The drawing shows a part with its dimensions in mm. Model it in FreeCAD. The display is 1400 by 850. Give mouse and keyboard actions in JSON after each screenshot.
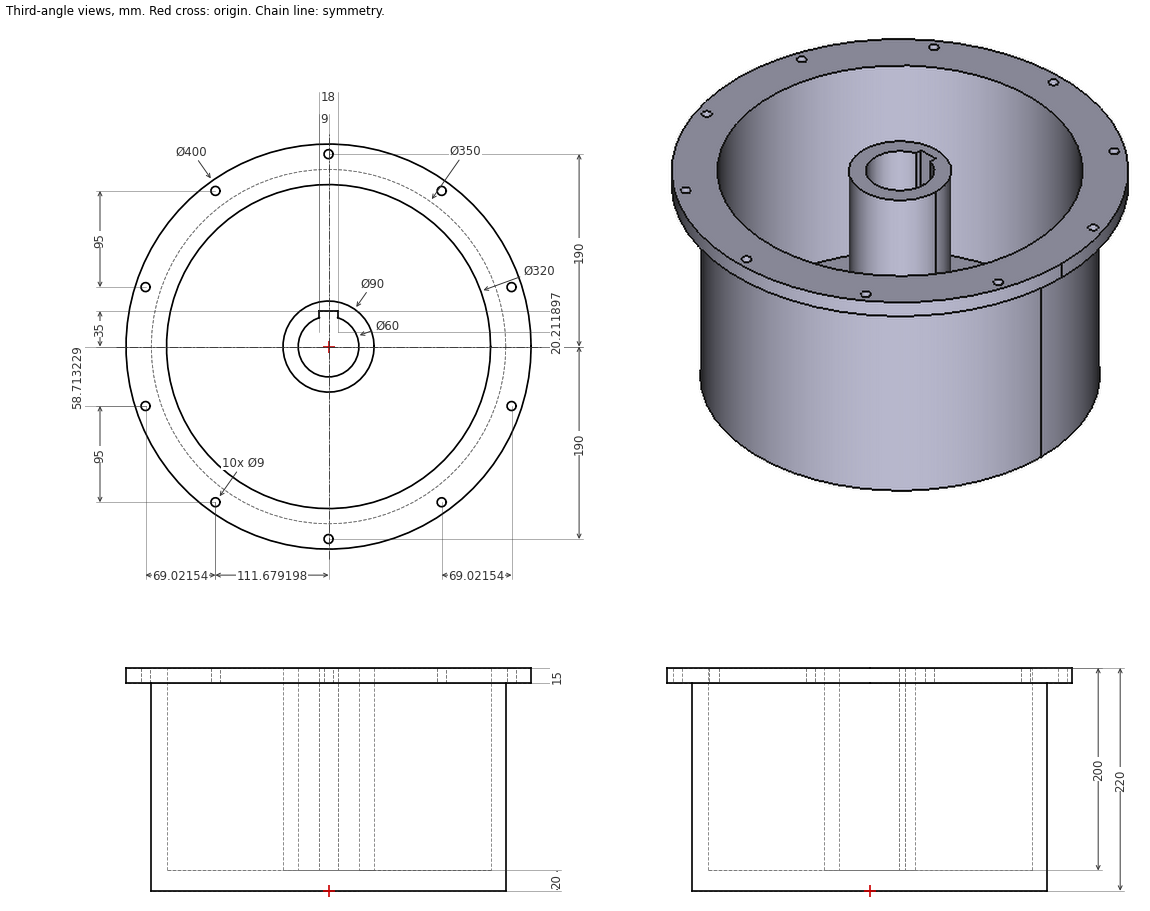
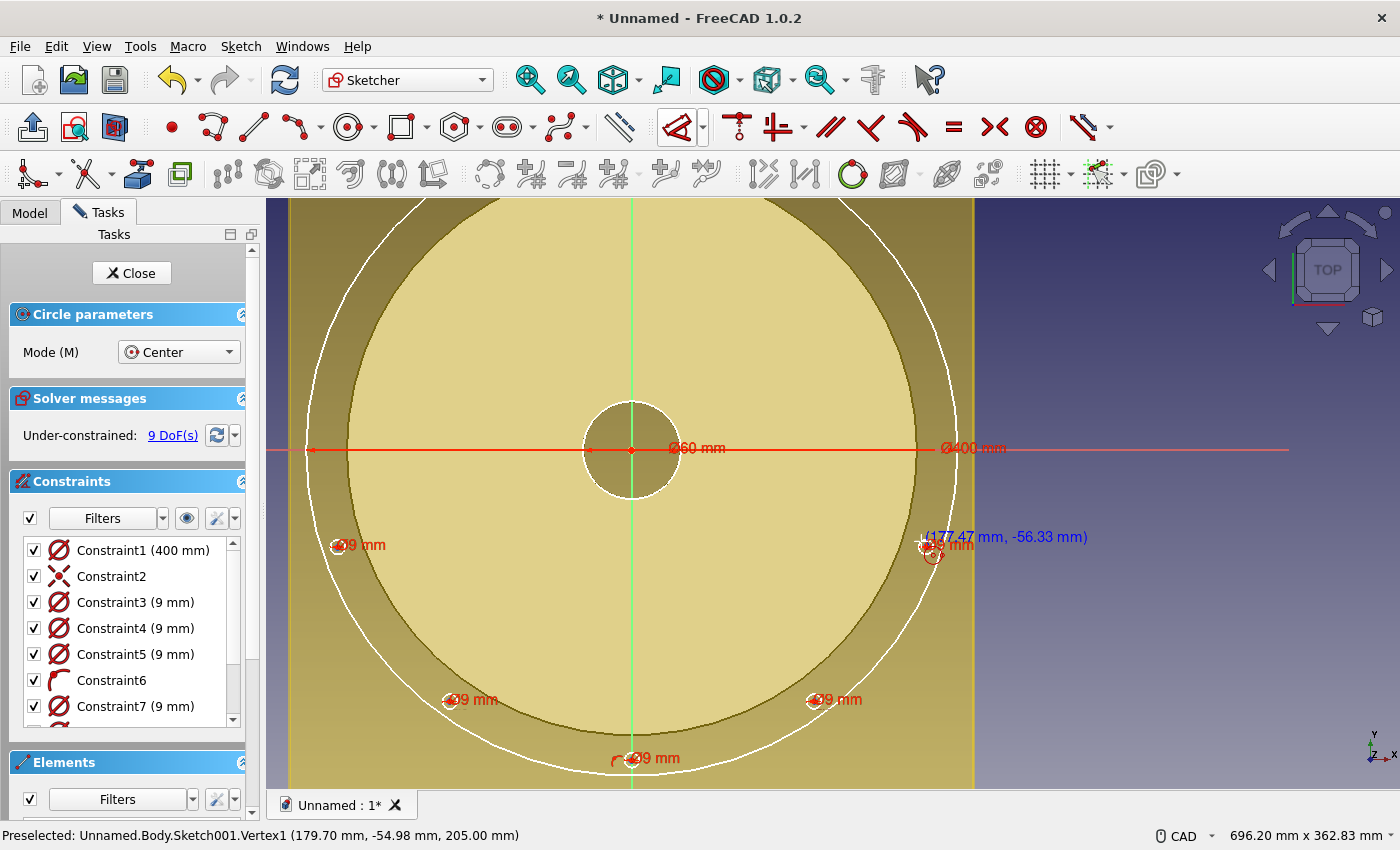
{"action": "scroll", "coordinate": [338, 355], "scroll_direction": "up", "scroll_amount": 6}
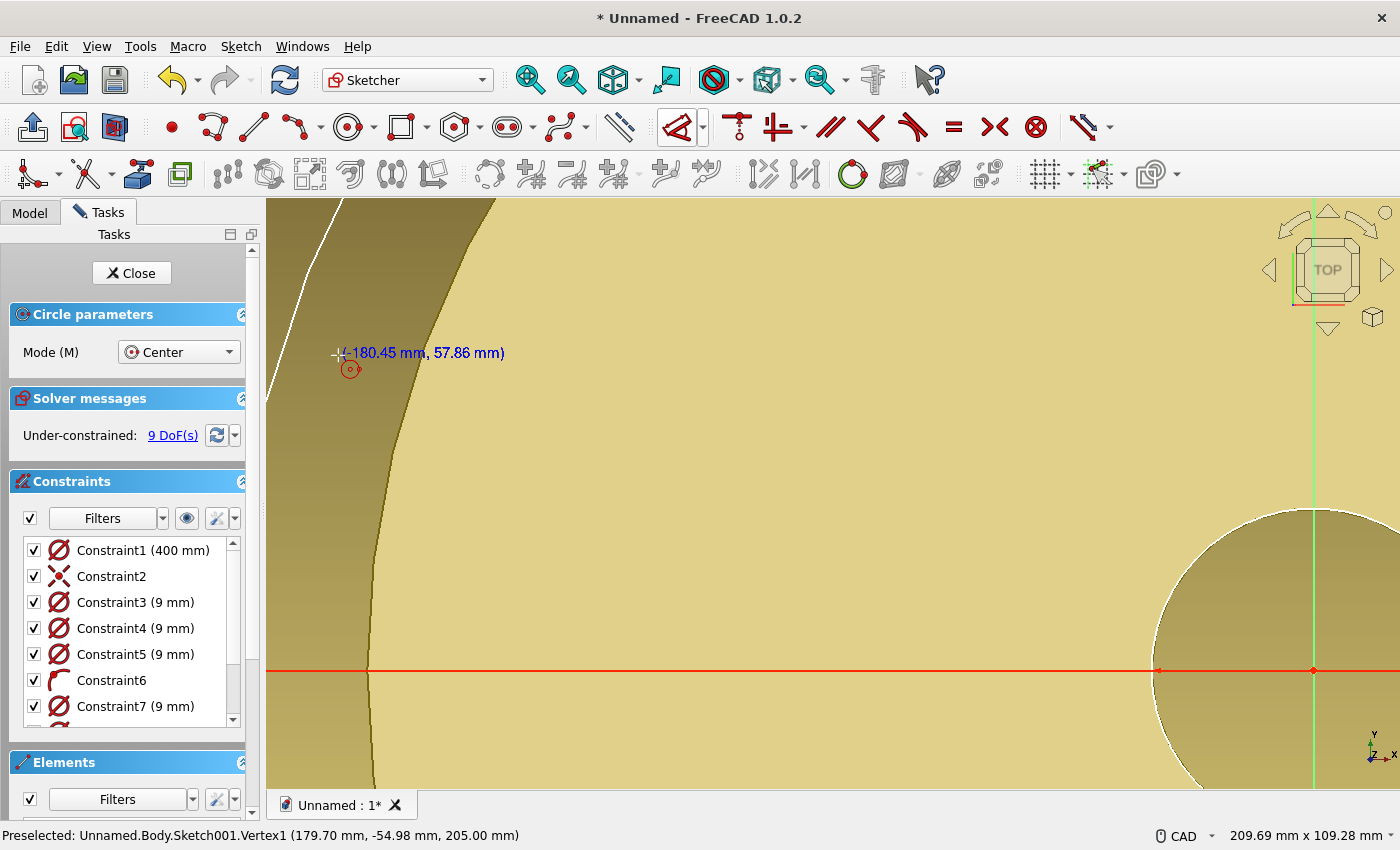
{"action": "scroll", "coordinate": [656, 458], "scroll_direction": "down", "scroll_amount": 9}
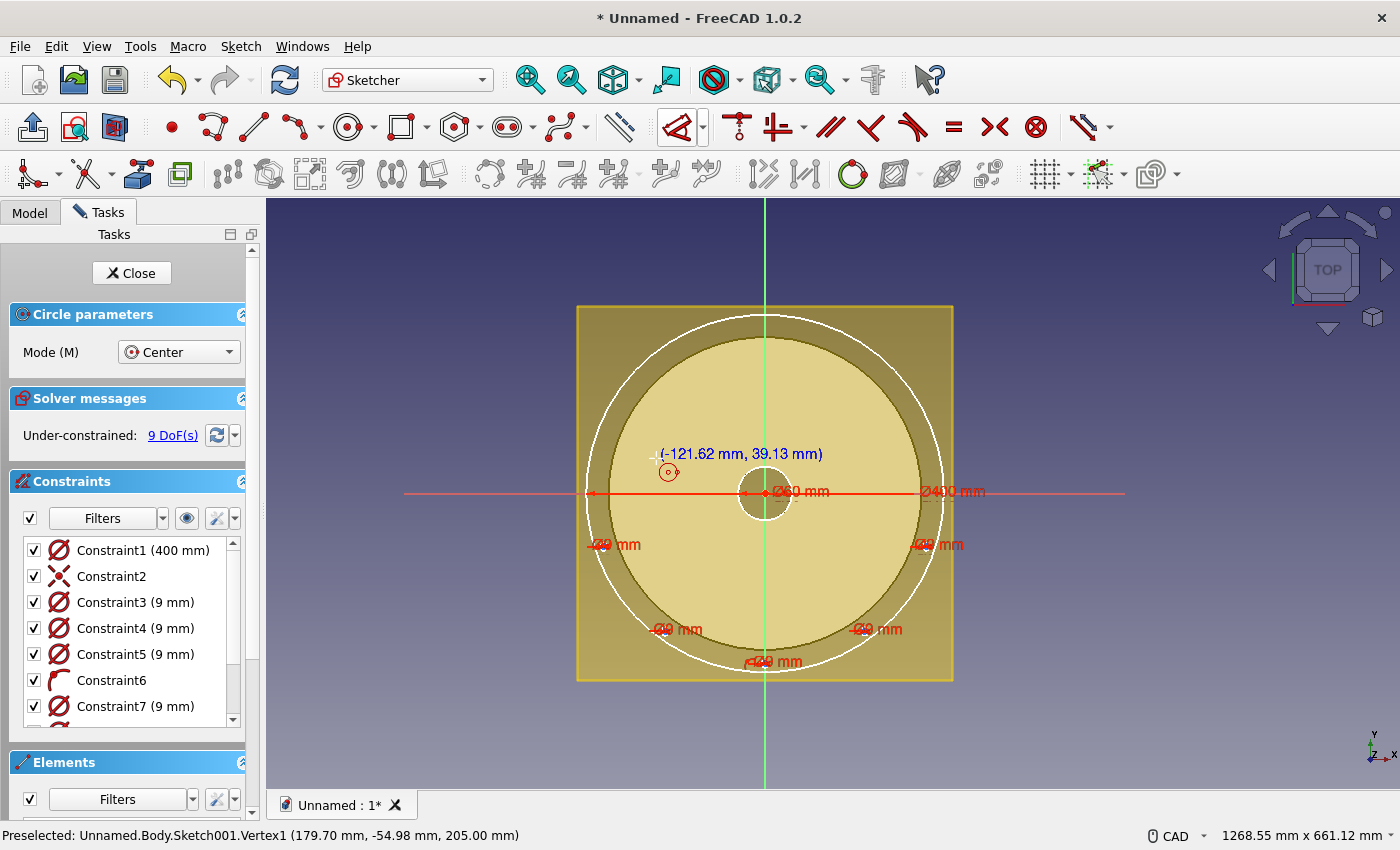
{"action": "scroll", "coordinate": [603, 441], "scroll_direction": "up", "scroll_amount": 3}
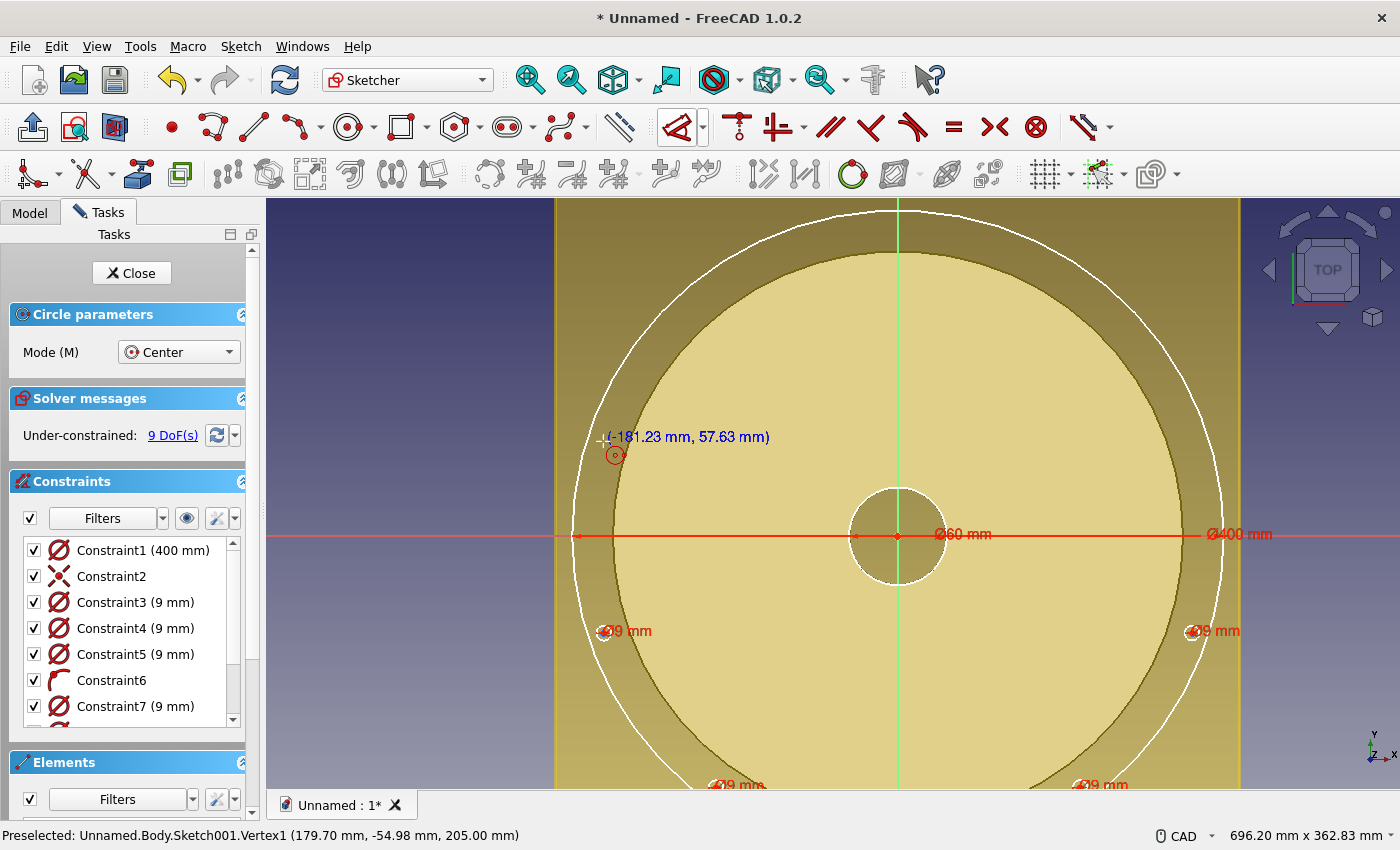
{"action": "left_click", "coordinate": [604, 441]}
{"action": "mouse_move", "coordinate": [609, 436]}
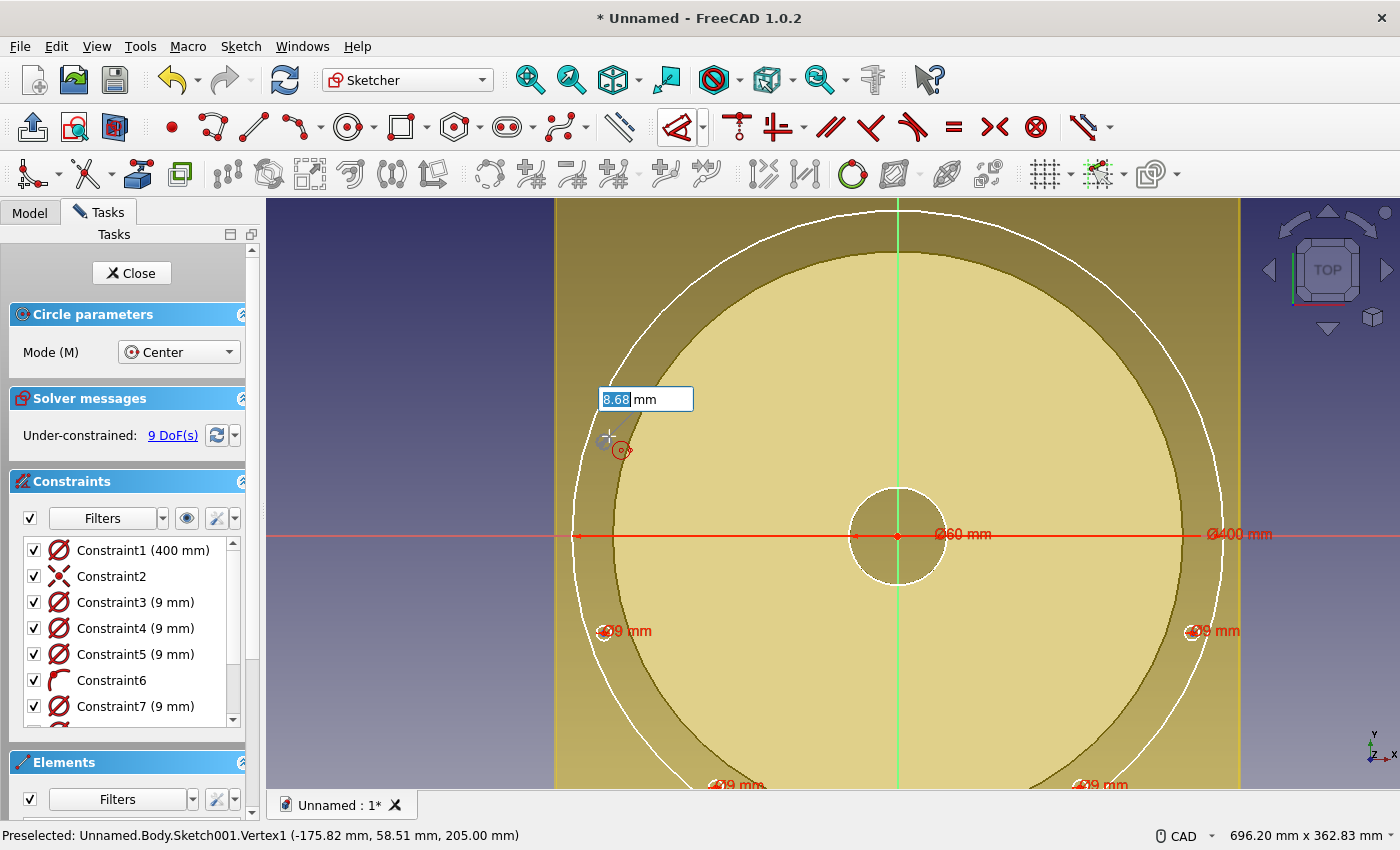
{"action": "type", "text": "9"}
{"action": "key", "text": "Return"}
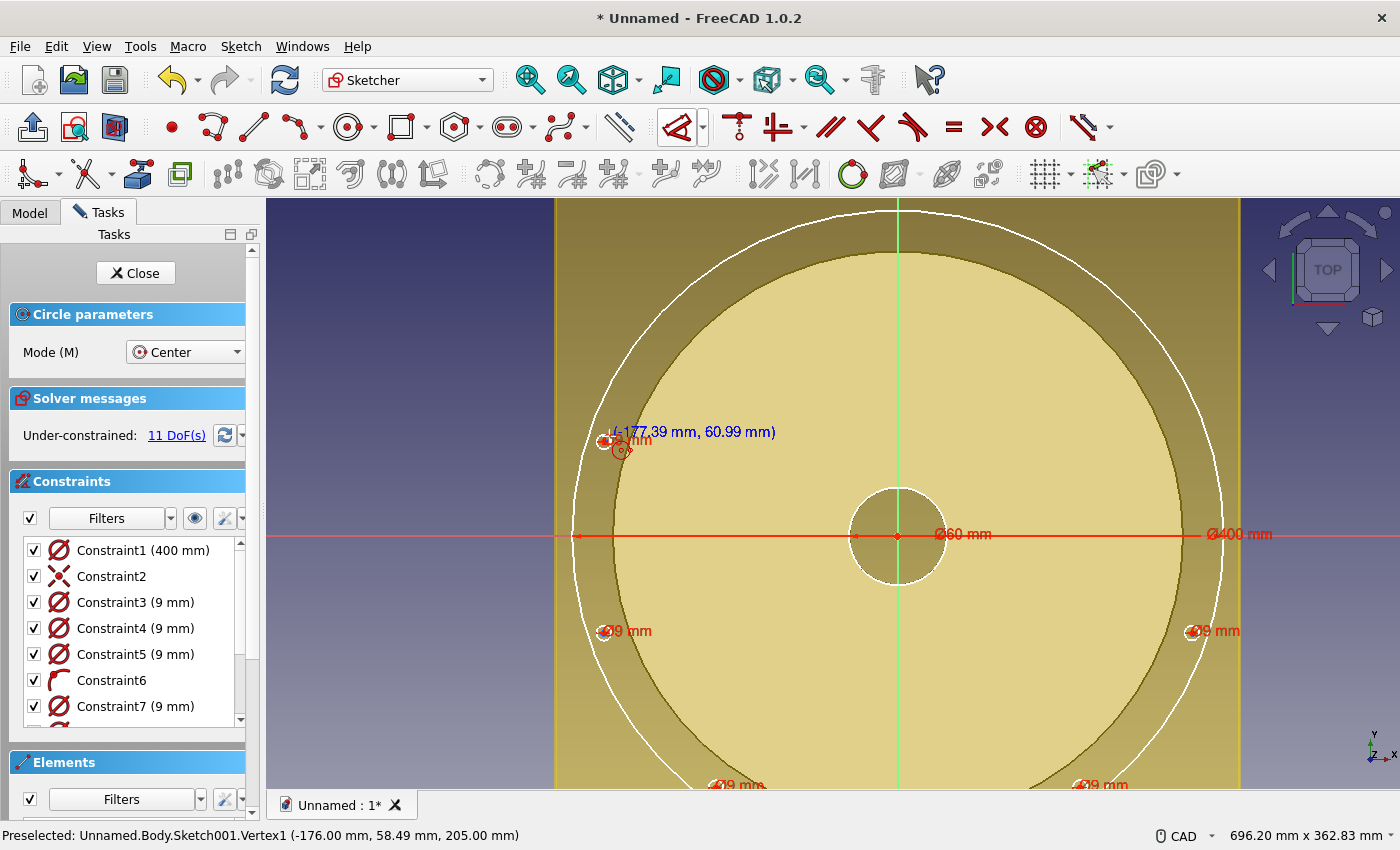
{"action": "scroll", "coordinate": [716, 286], "scroll_direction": "up", "scroll_amount": 6}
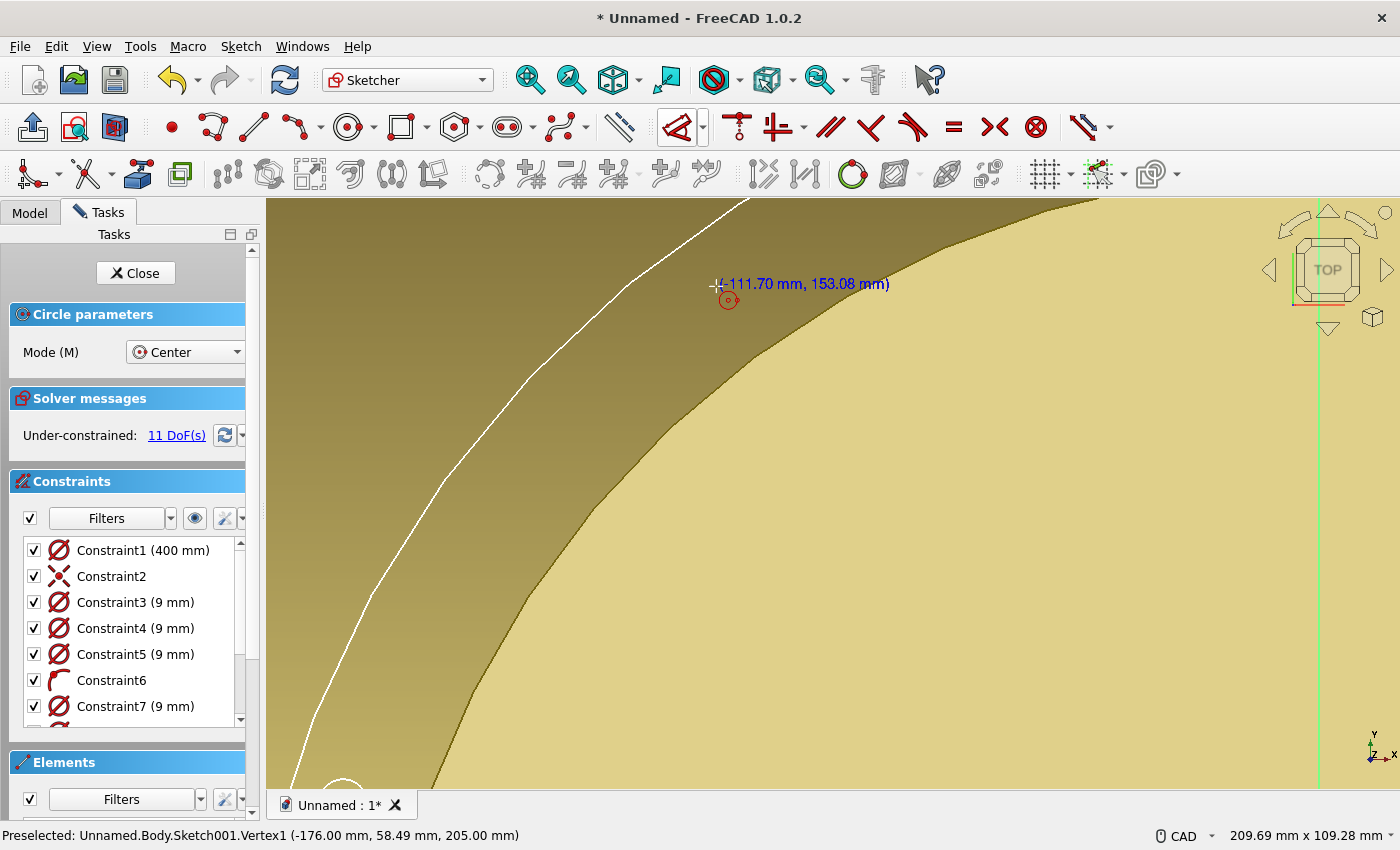
{"action": "scroll", "coordinate": [655, 370], "scroll_direction": "down", "scroll_amount": 9}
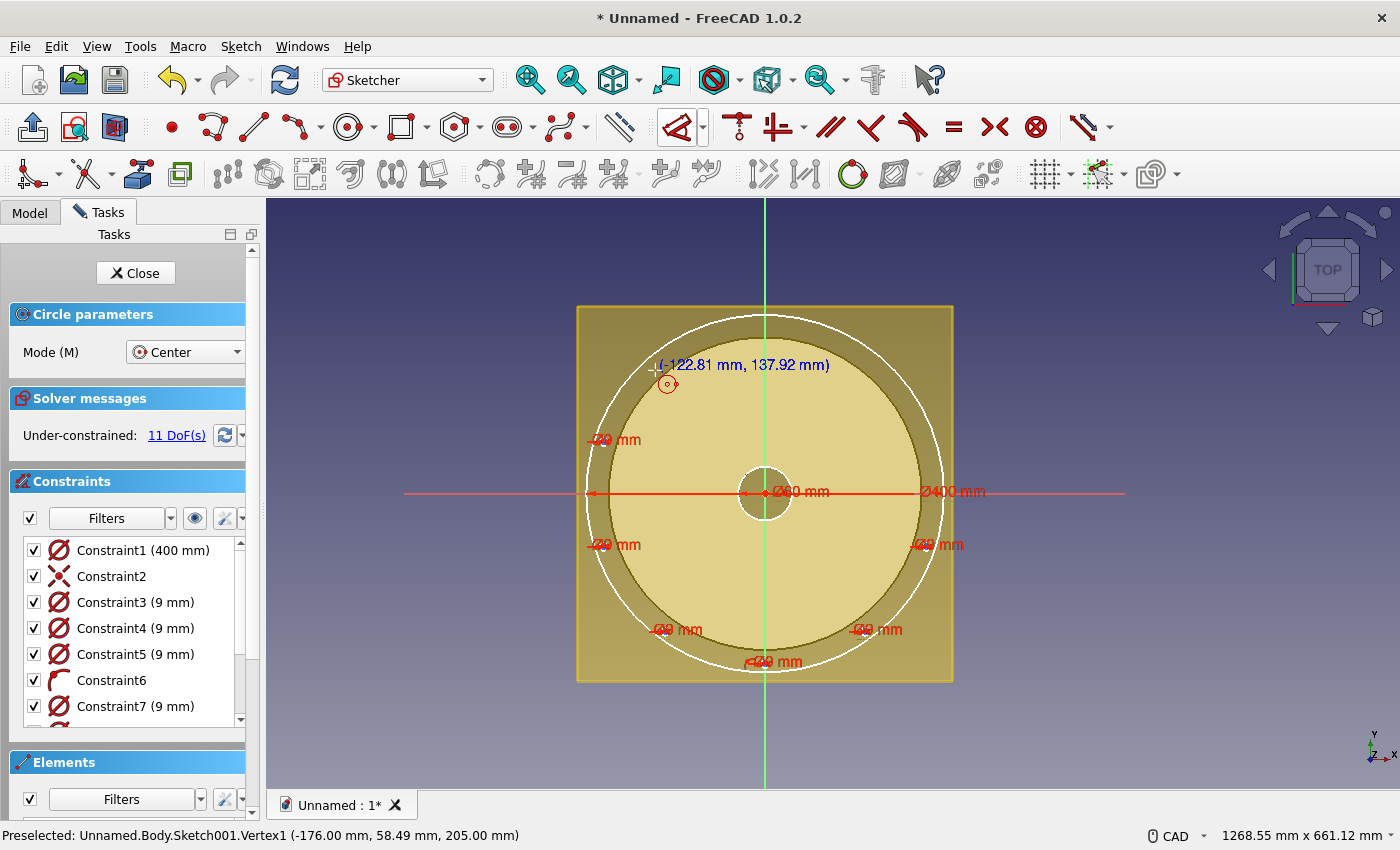
{"action": "scroll", "coordinate": [665, 356], "scroll_direction": "up", "scroll_amount": 3}